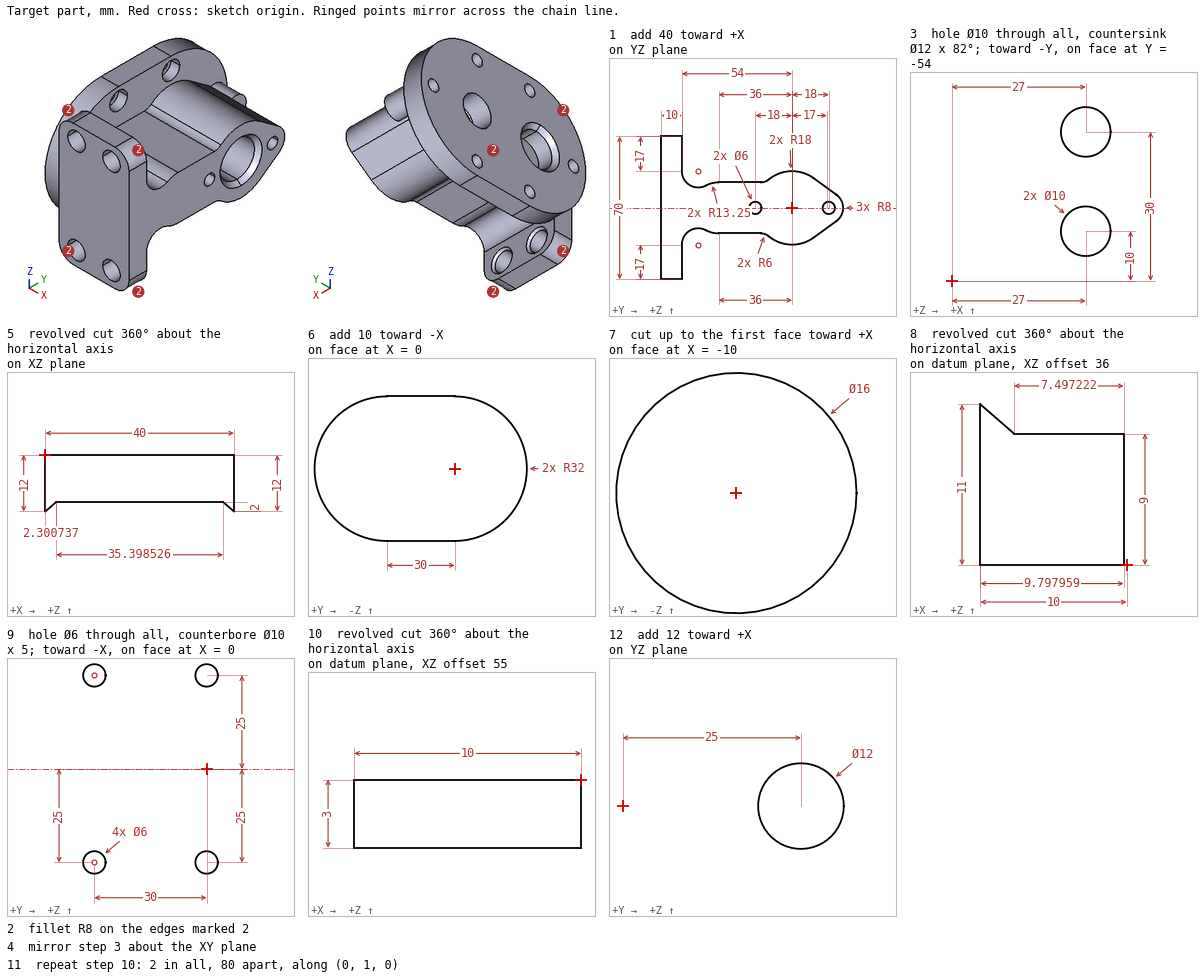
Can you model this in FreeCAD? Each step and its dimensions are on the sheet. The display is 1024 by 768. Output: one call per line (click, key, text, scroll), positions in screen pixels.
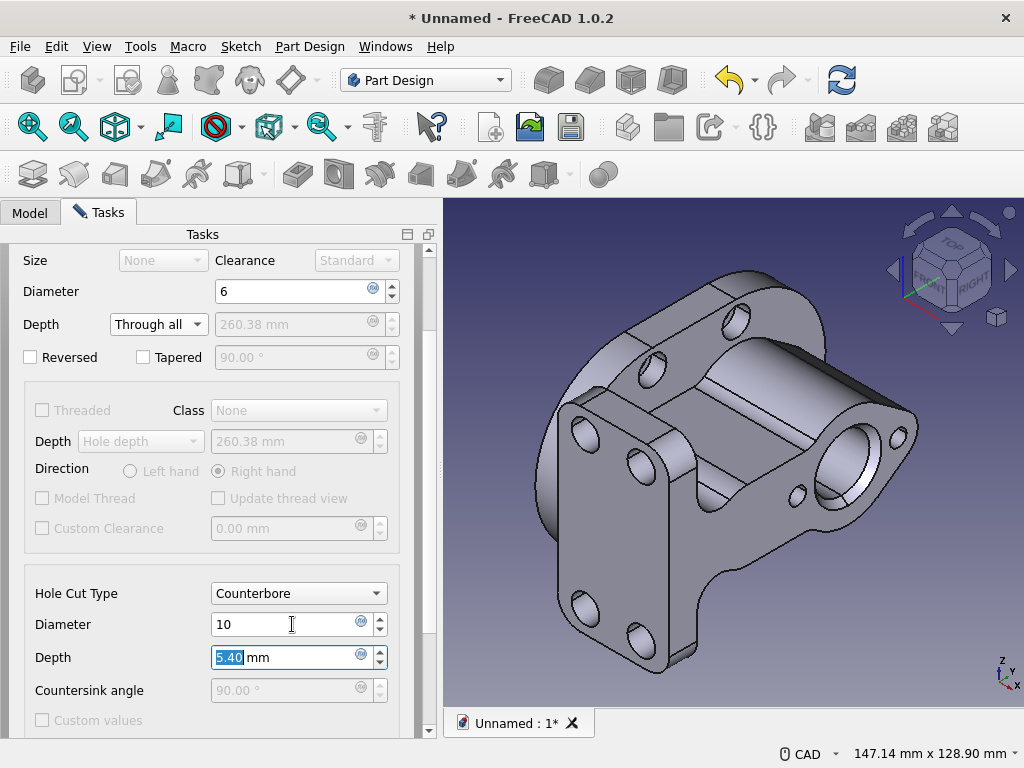
text(5)
key(Tab)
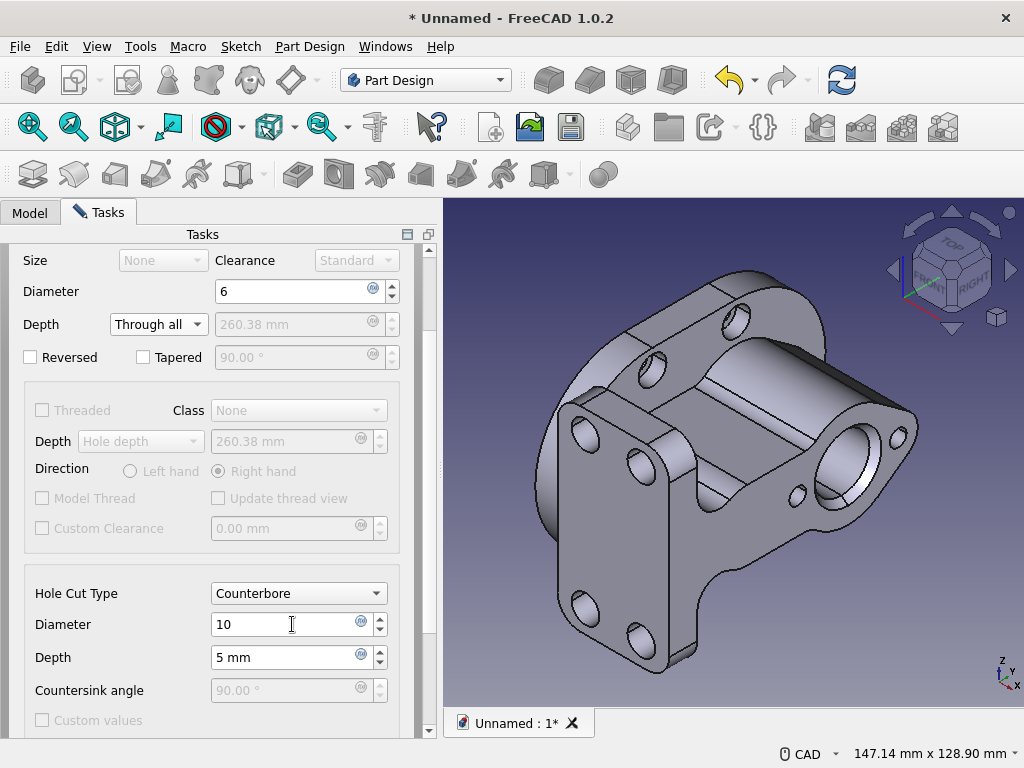
scroll(429, 491, up, 3)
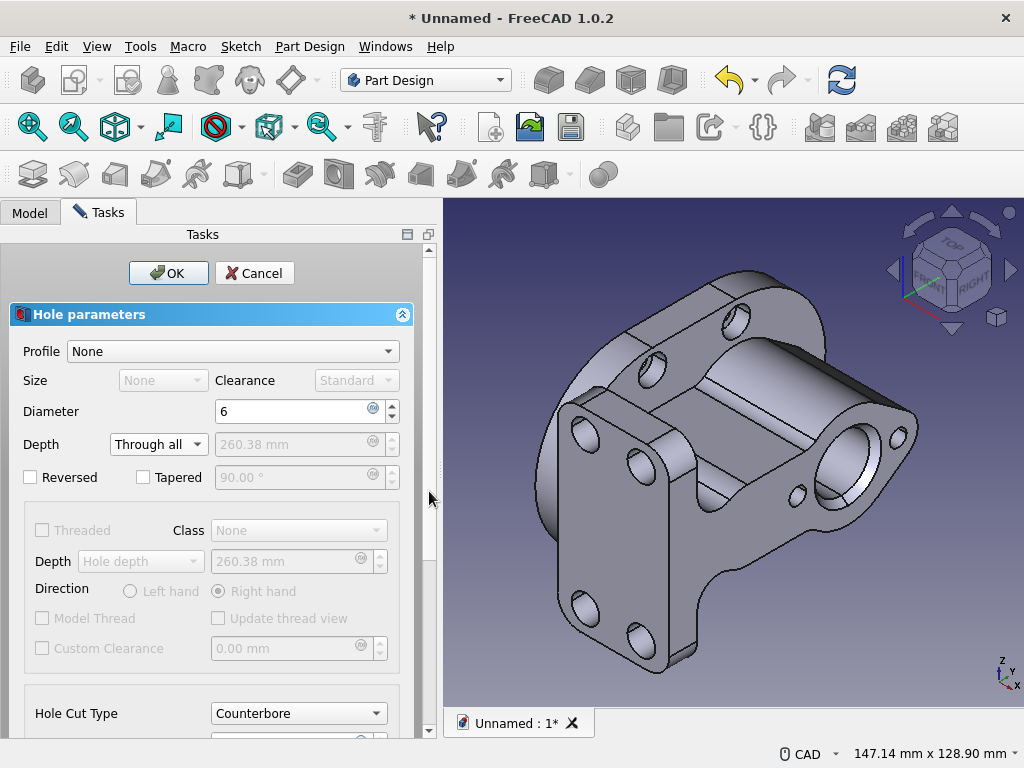
click(169, 273)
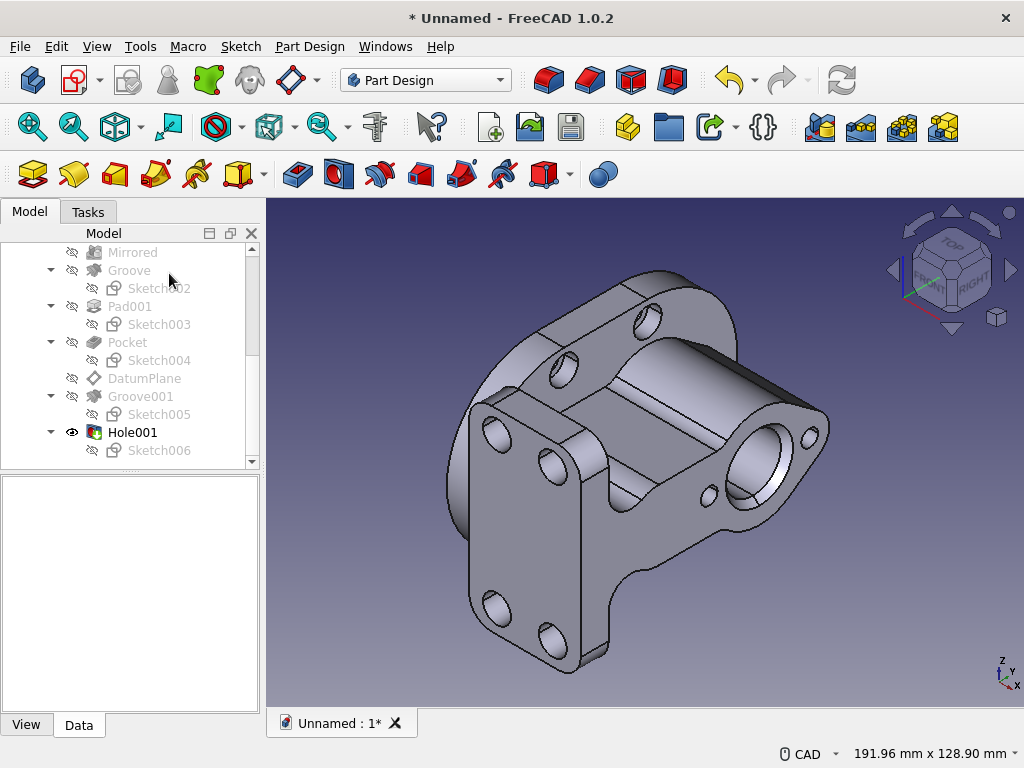
scroll(141, 356, down, 3)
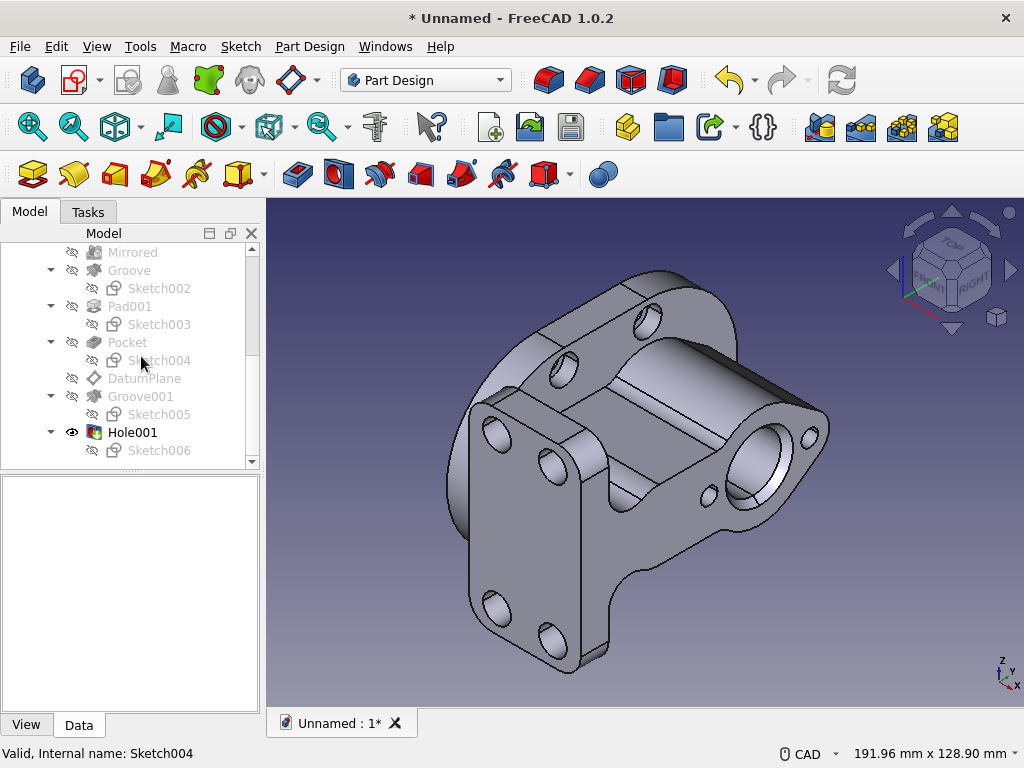
scroll(141, 356, up, 15)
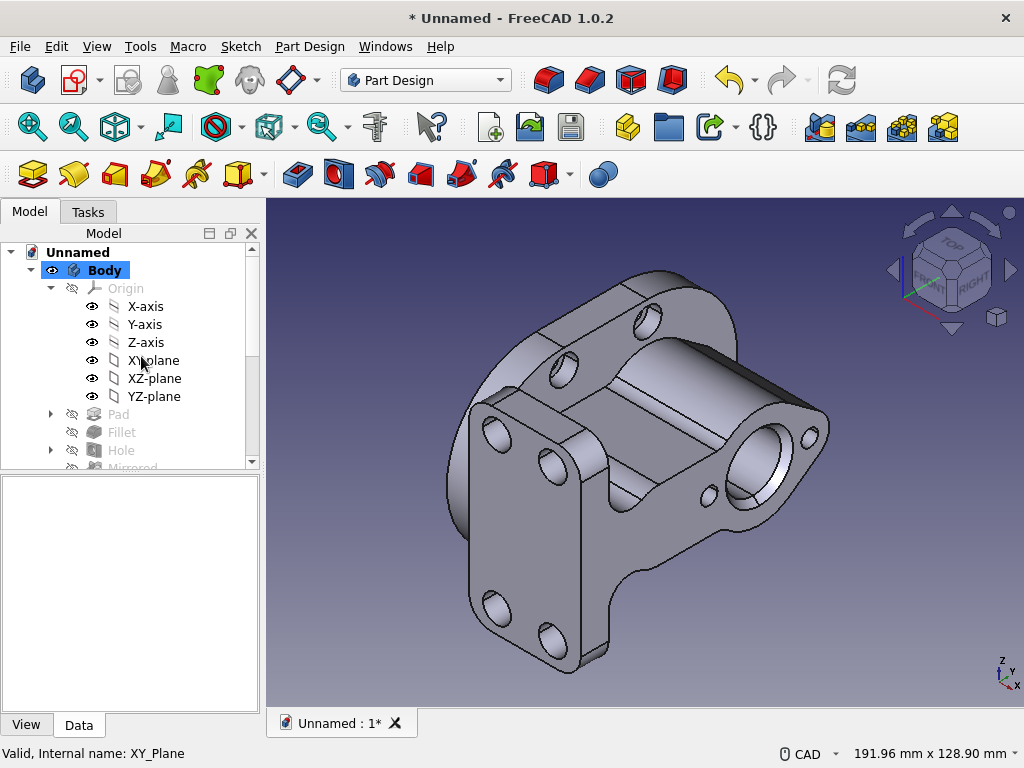
click(137, 378)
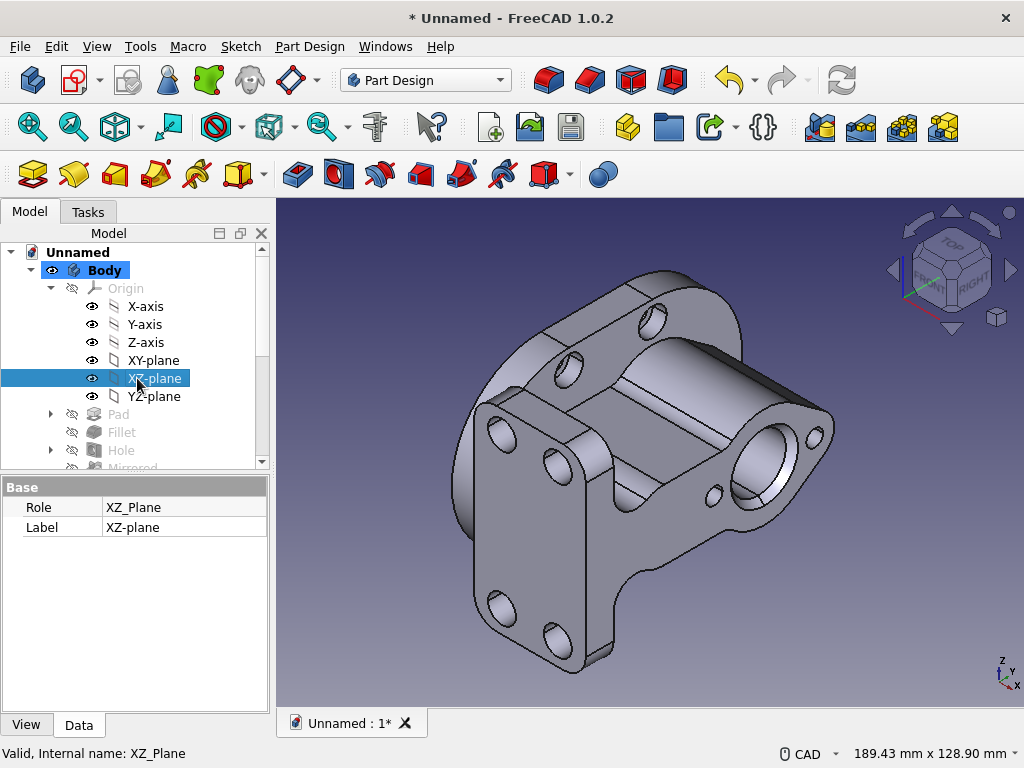
click(290, 80)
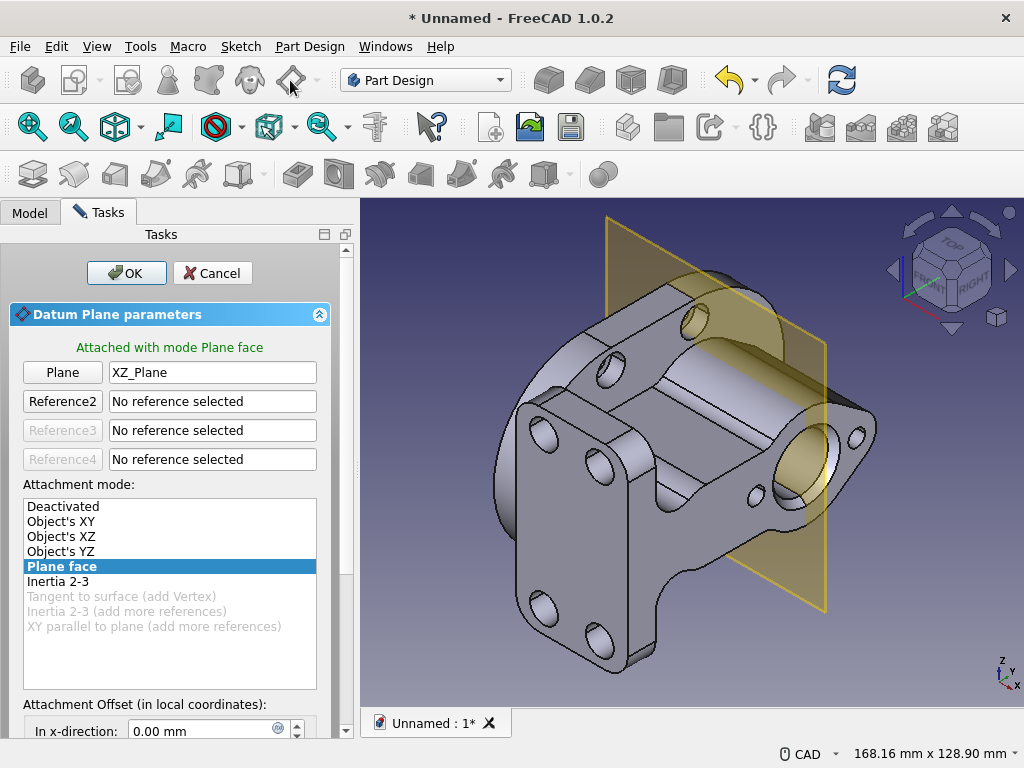
scroll(346, 491, down, 3)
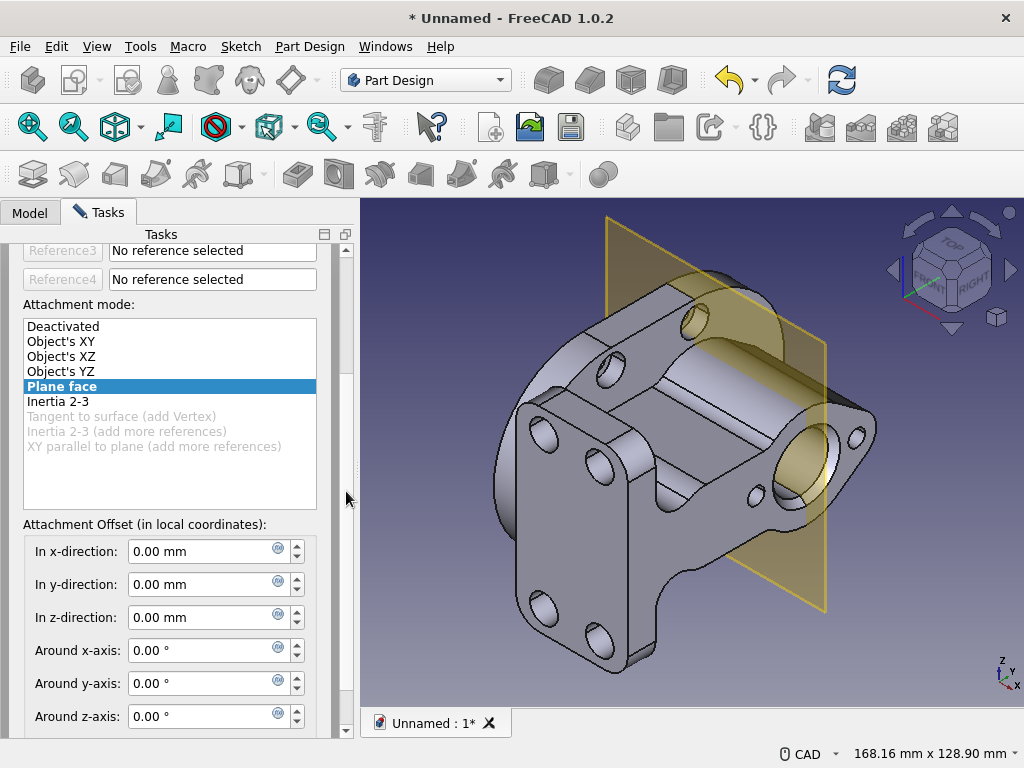
triple_click(210, 618)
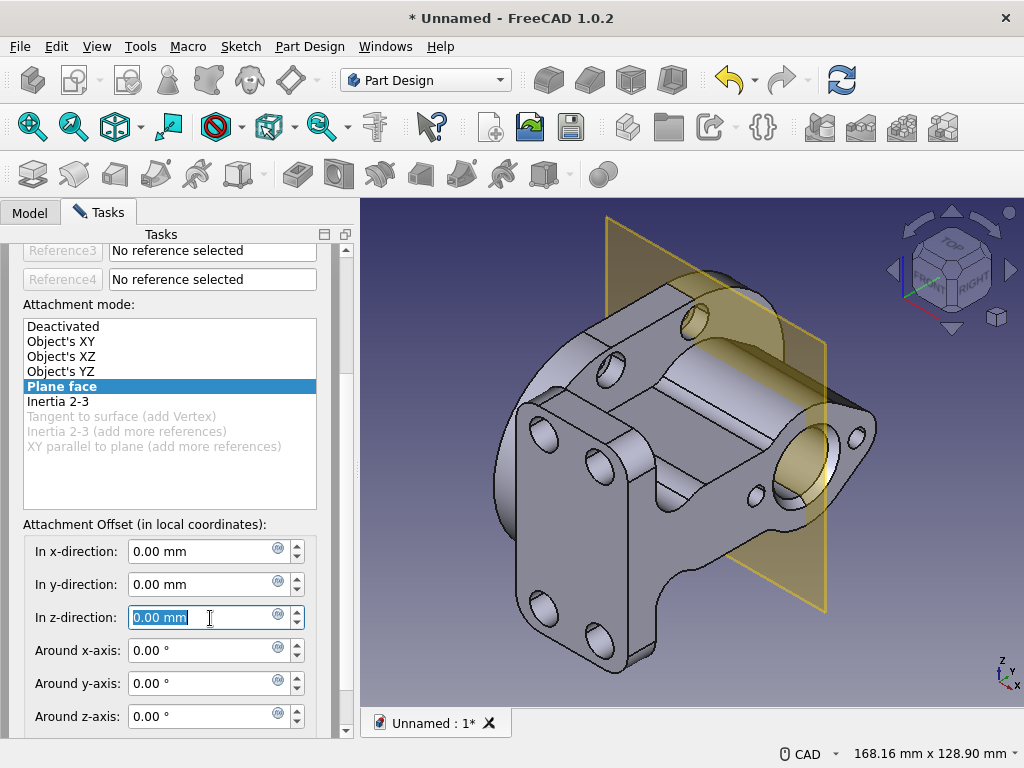
text(55)
key(Tab)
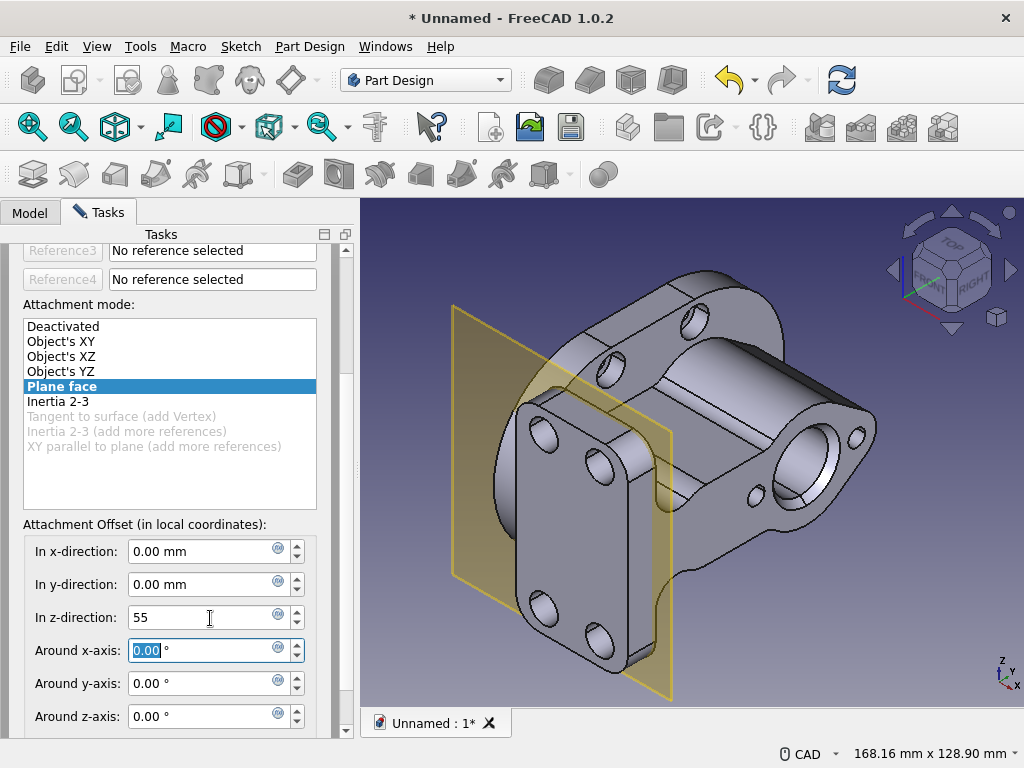
scroll(346, 491, up, 4)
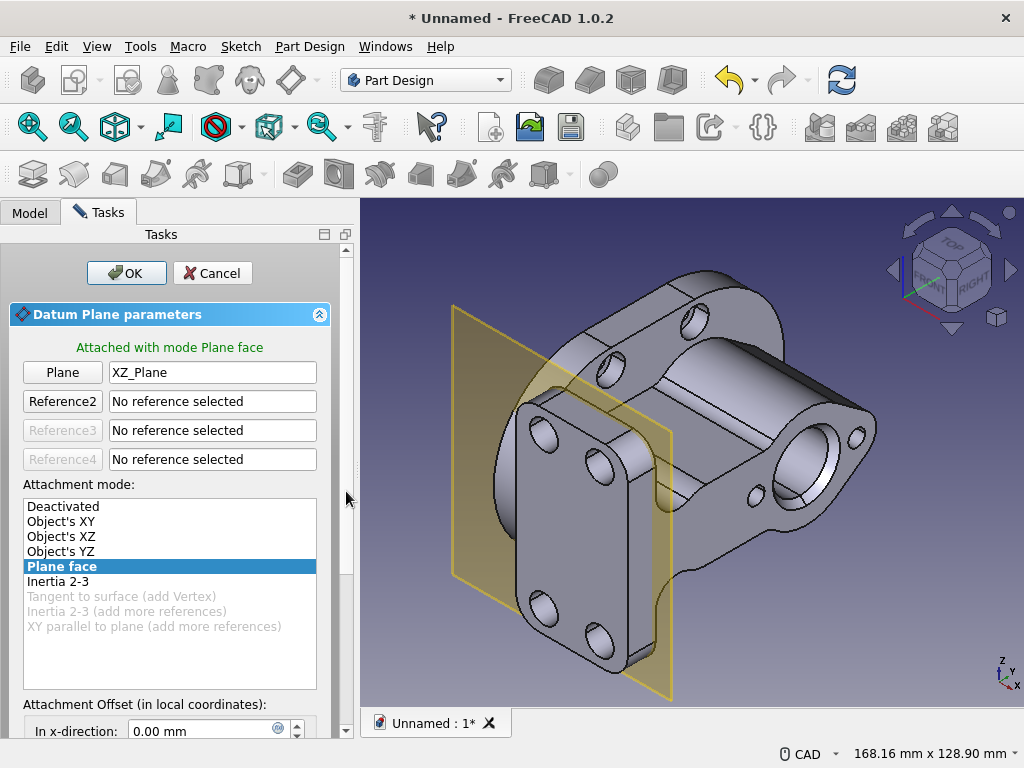
click(127, 273)